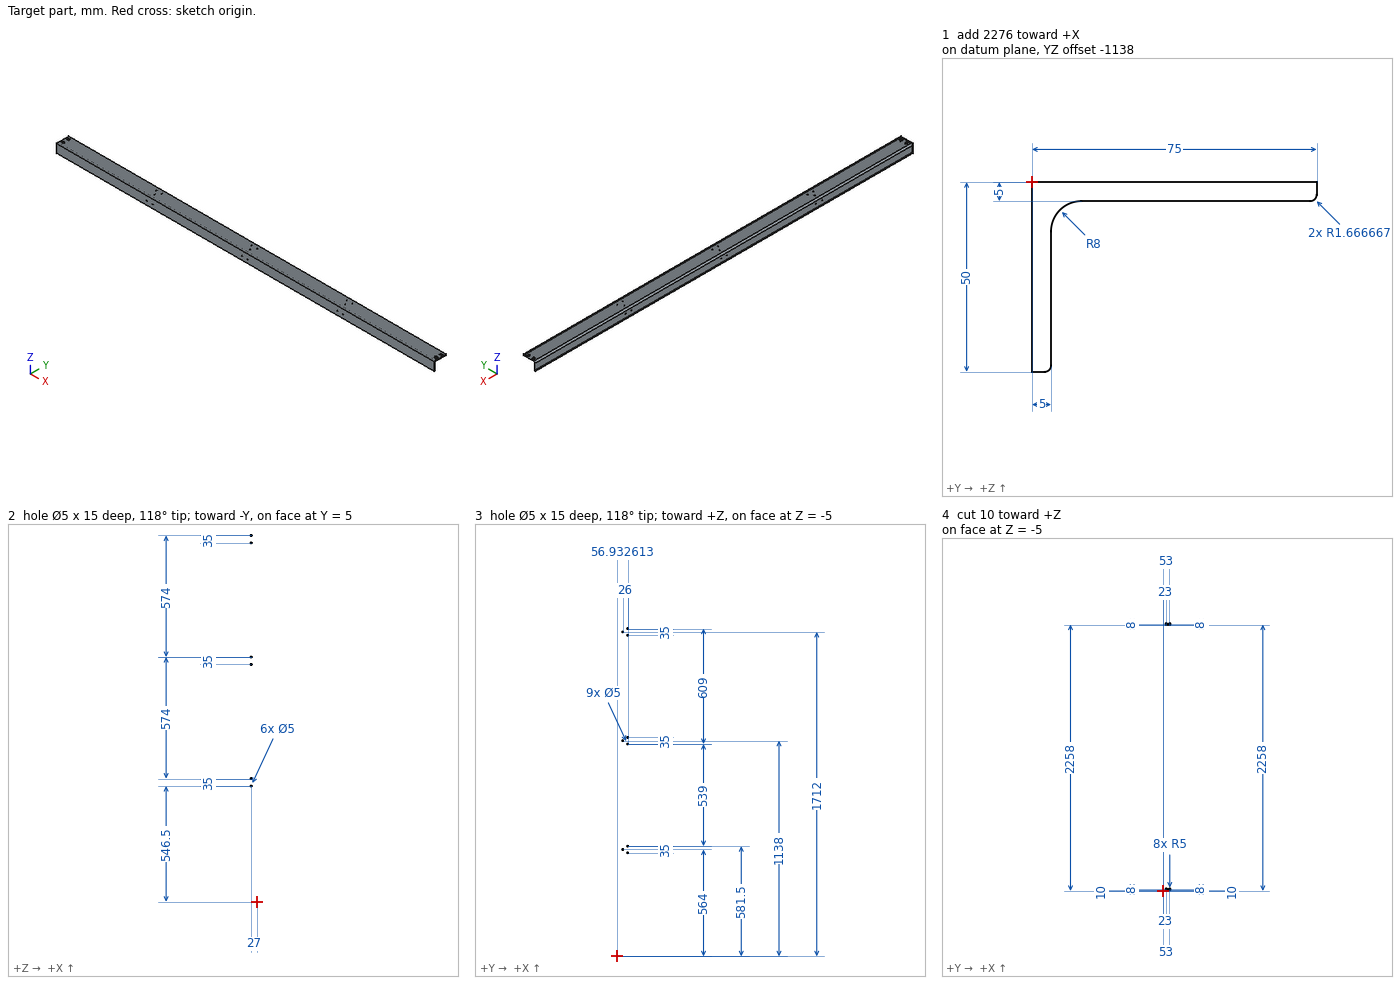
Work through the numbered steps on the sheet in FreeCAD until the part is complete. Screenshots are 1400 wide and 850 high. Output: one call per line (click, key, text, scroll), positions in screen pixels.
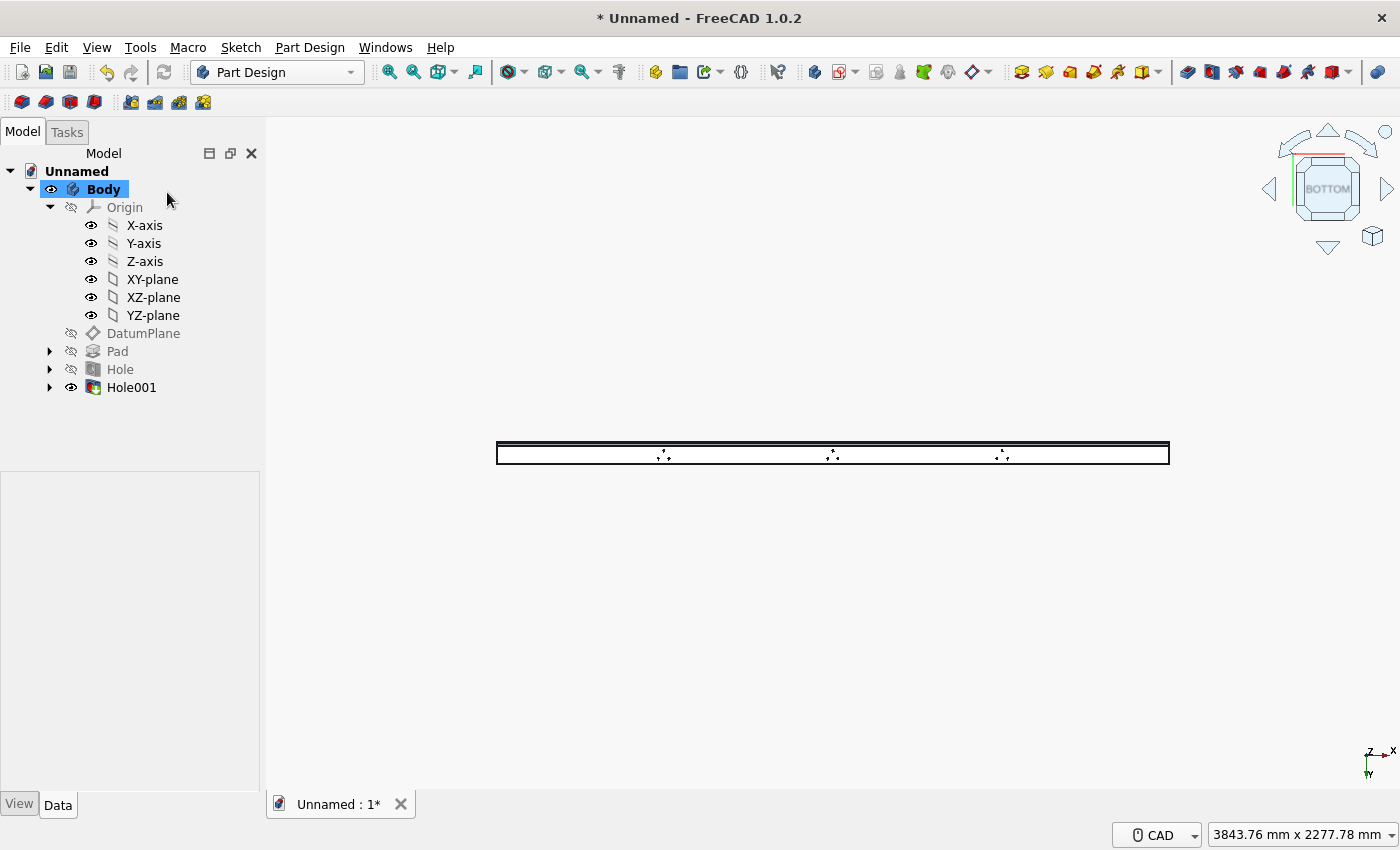
click(929, 454)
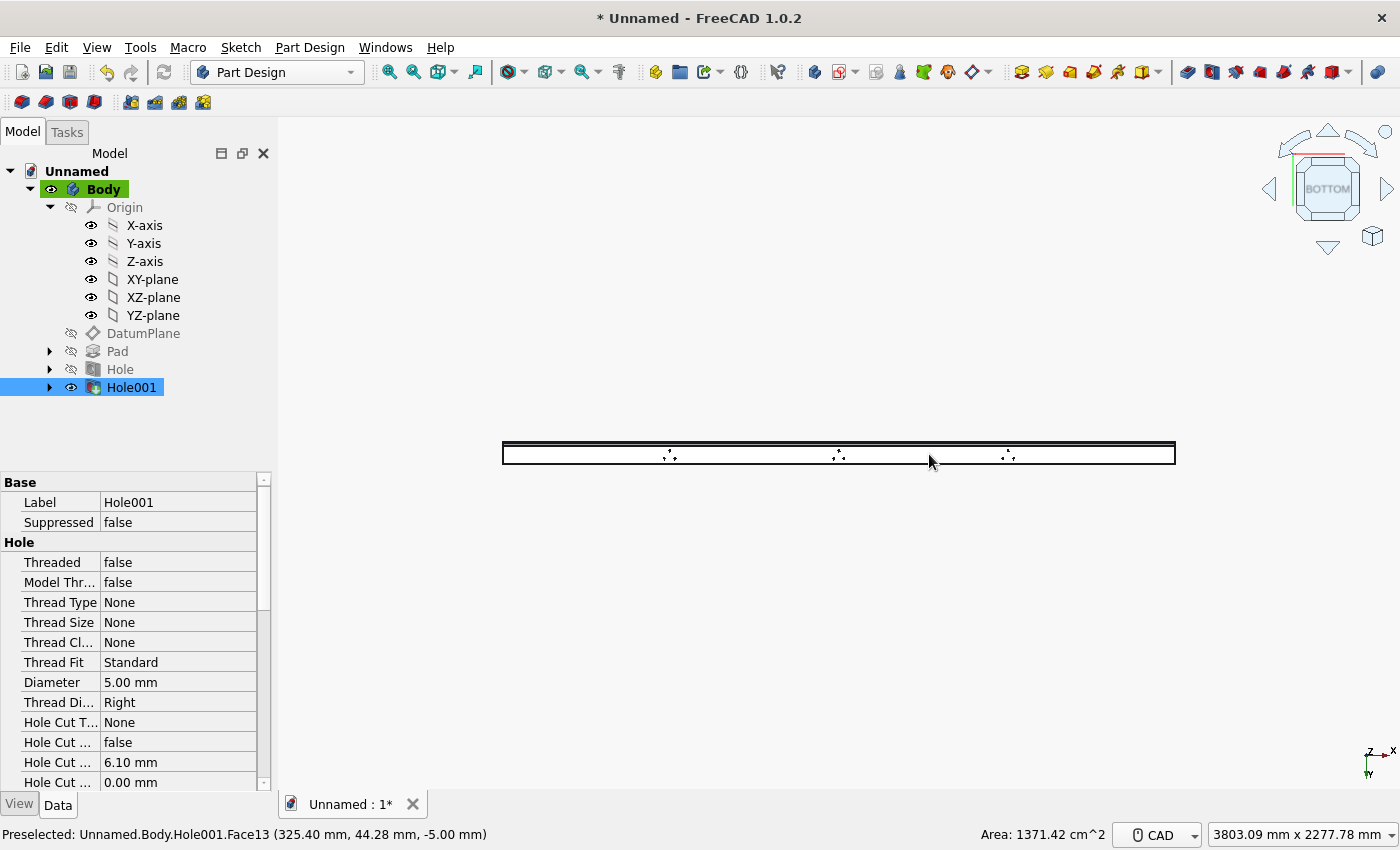
click(840, 72)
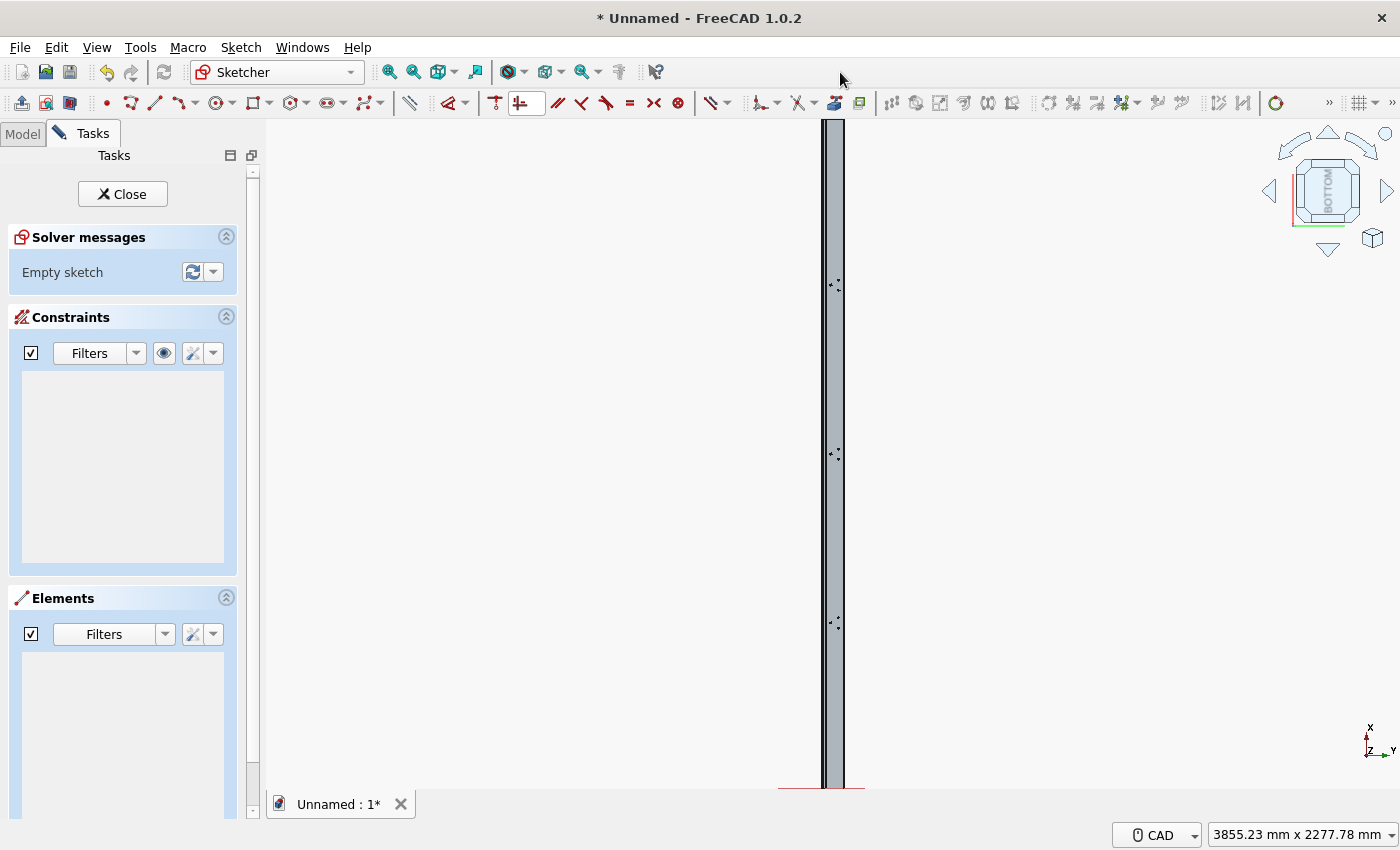
scroll(629, 453, down, 2)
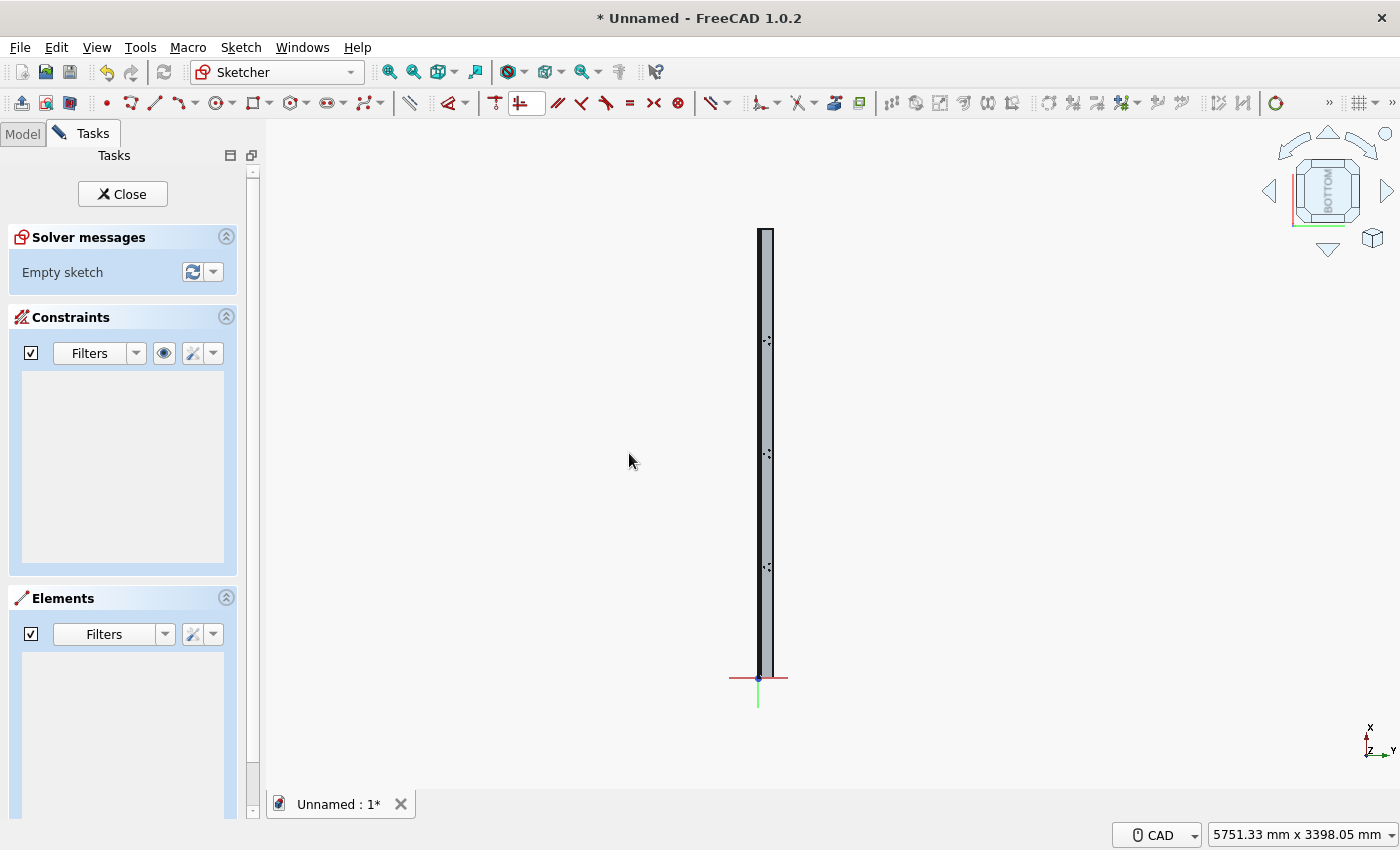
click(328, 104)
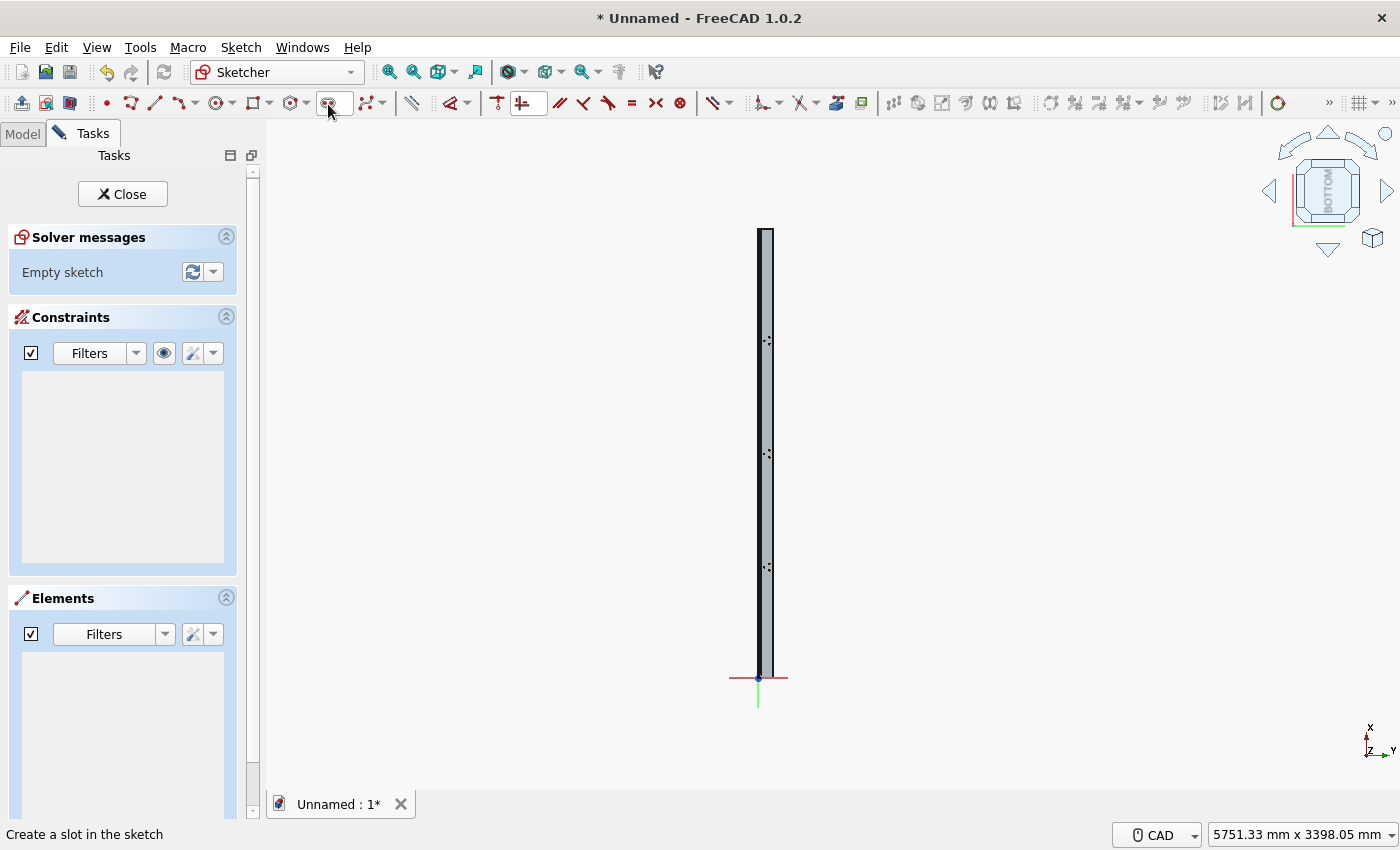
scroll(770, 676, up, 16)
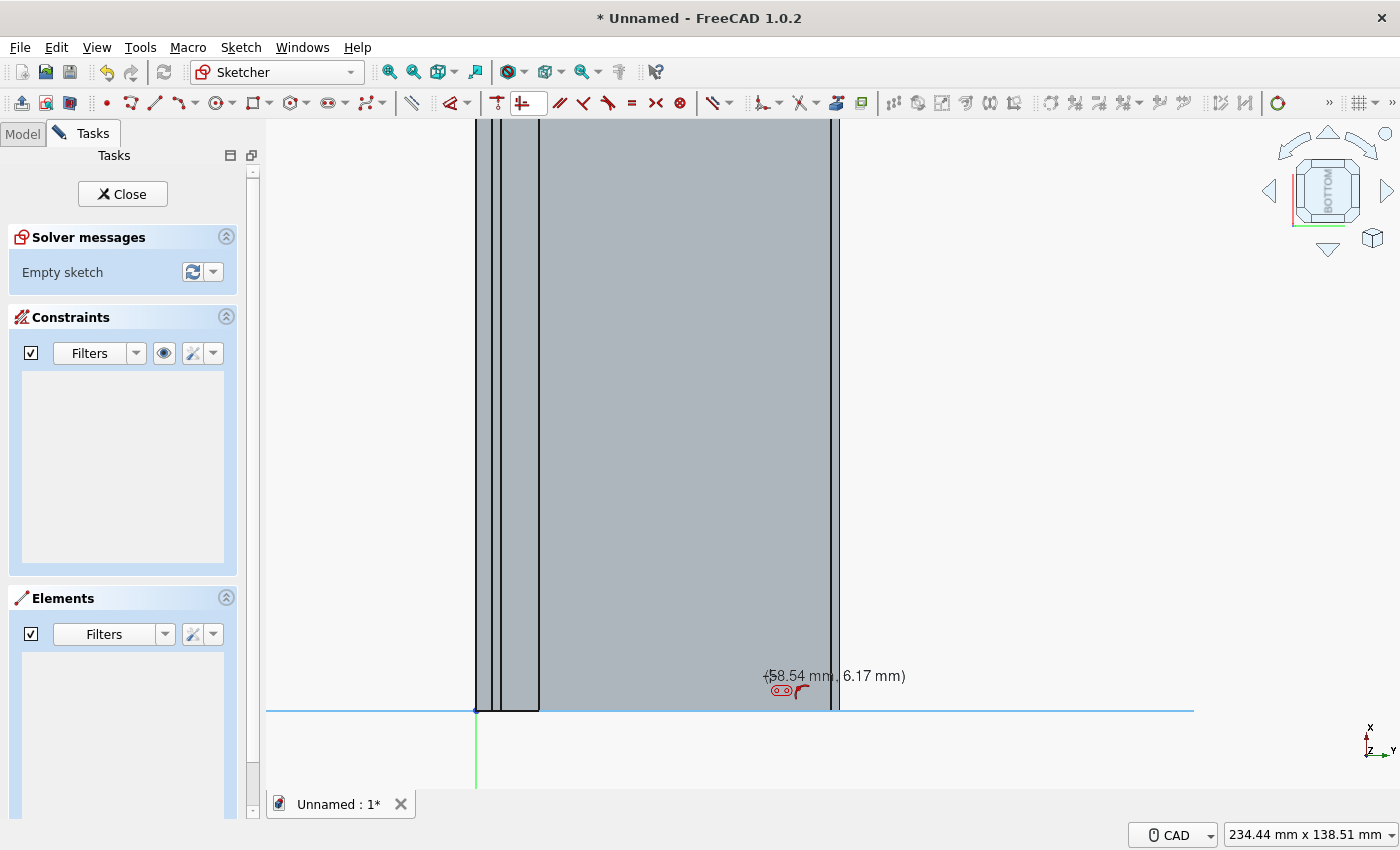
scroll(772, 728, down, 15)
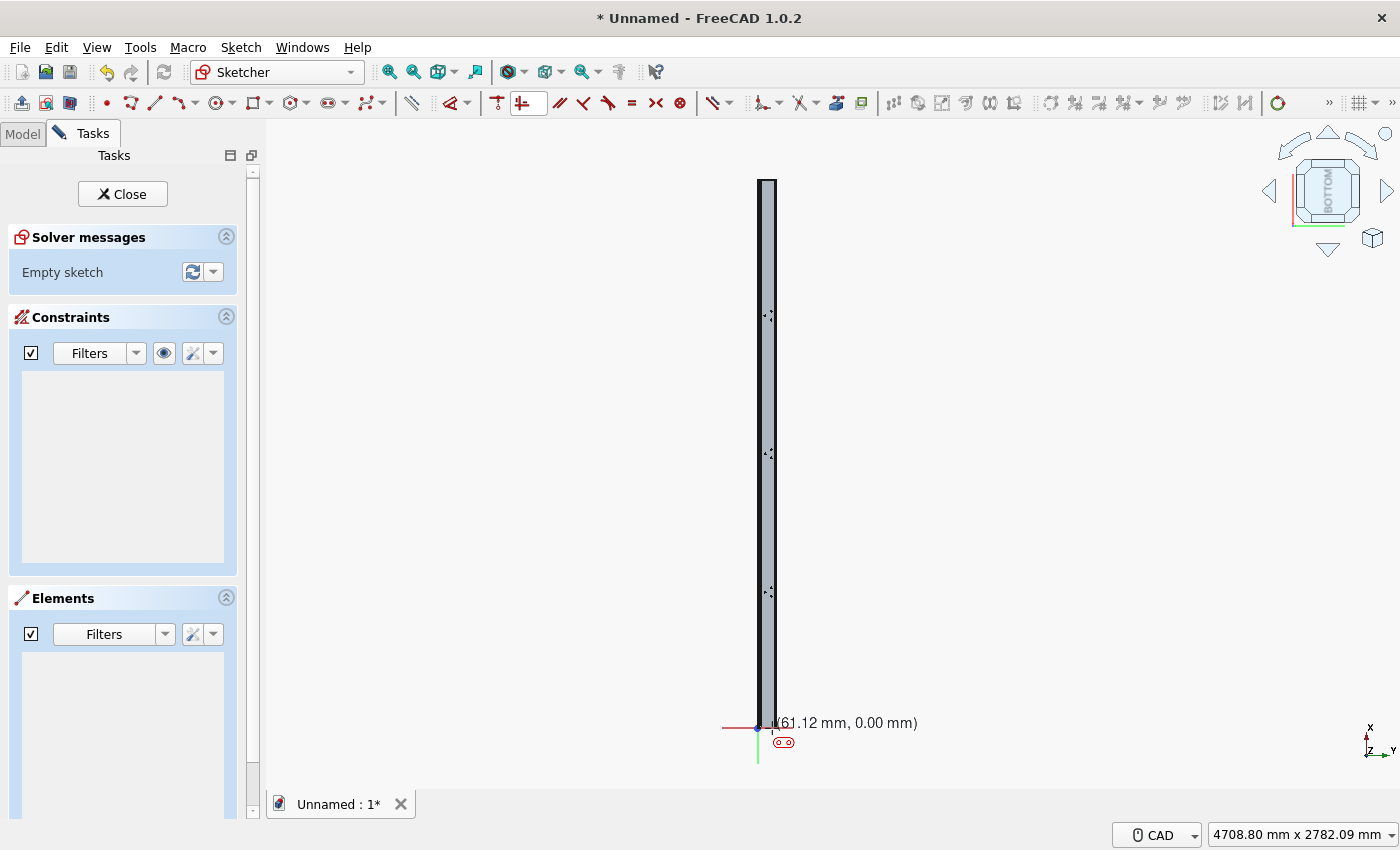
scroll(772, 726, up, 10)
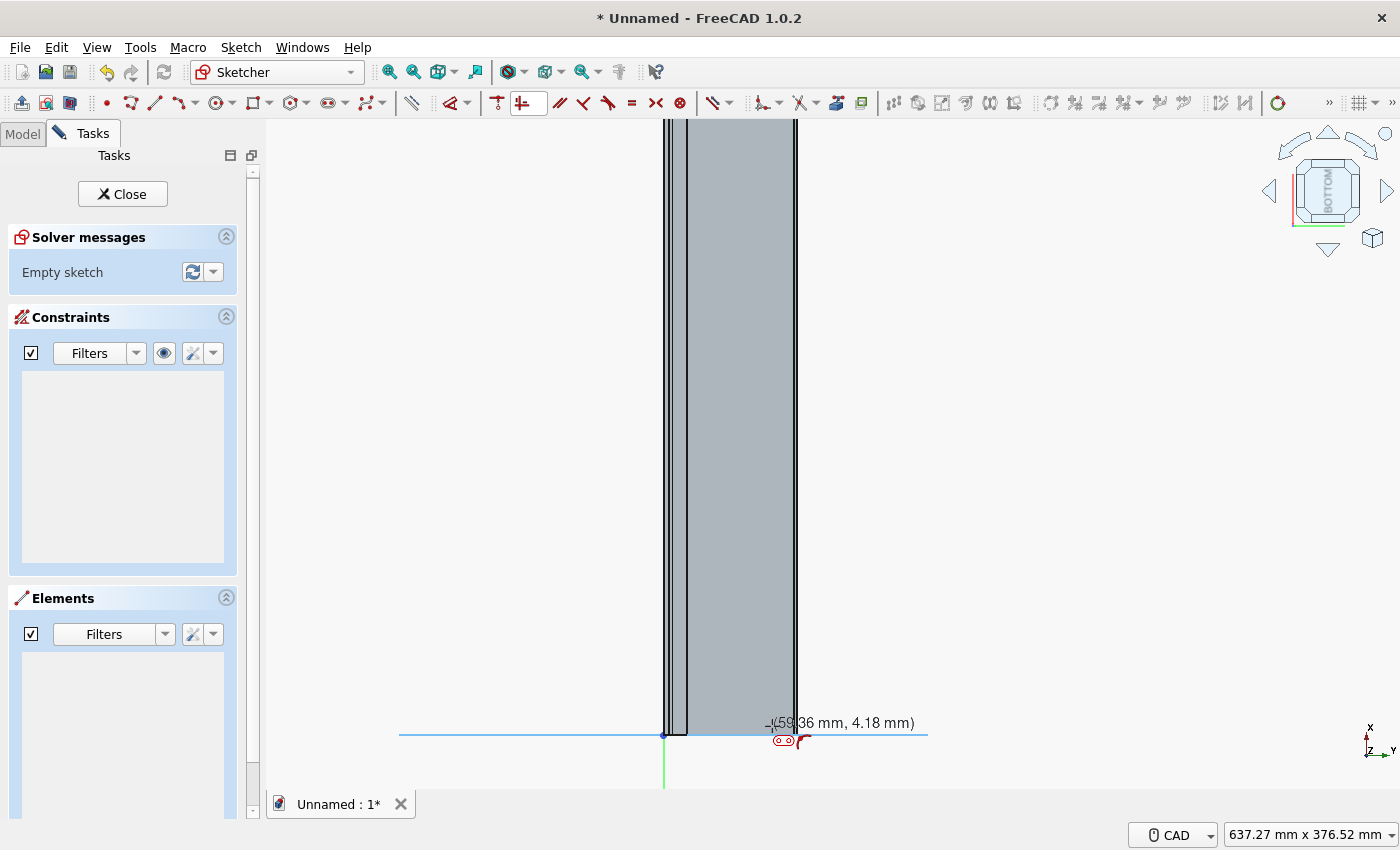
click(767, 717)